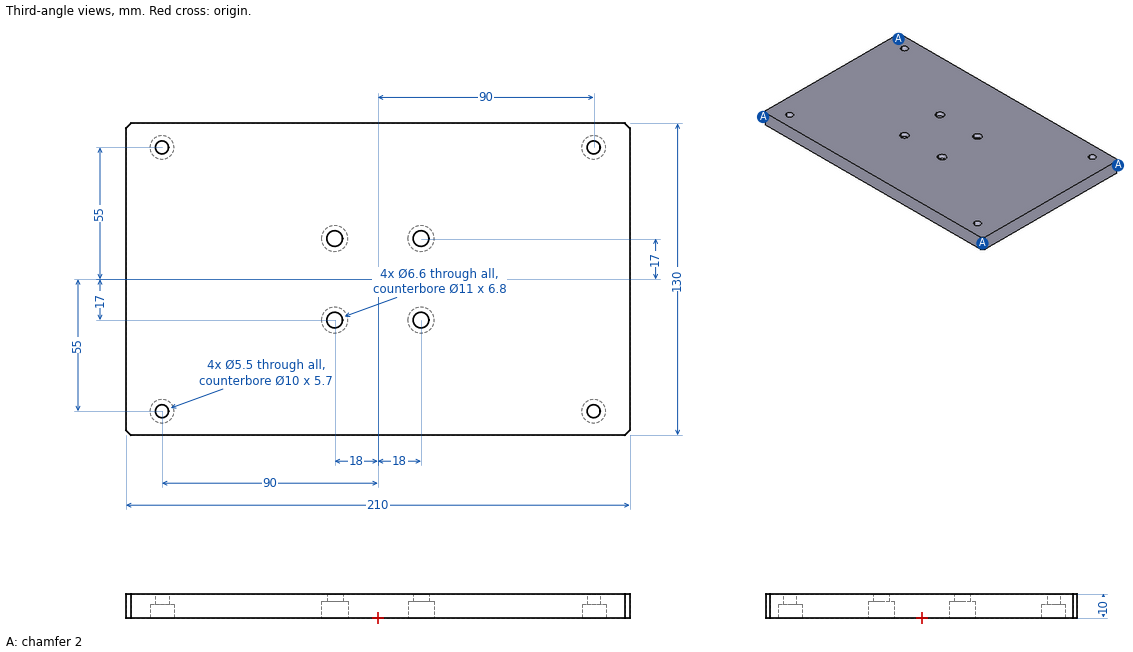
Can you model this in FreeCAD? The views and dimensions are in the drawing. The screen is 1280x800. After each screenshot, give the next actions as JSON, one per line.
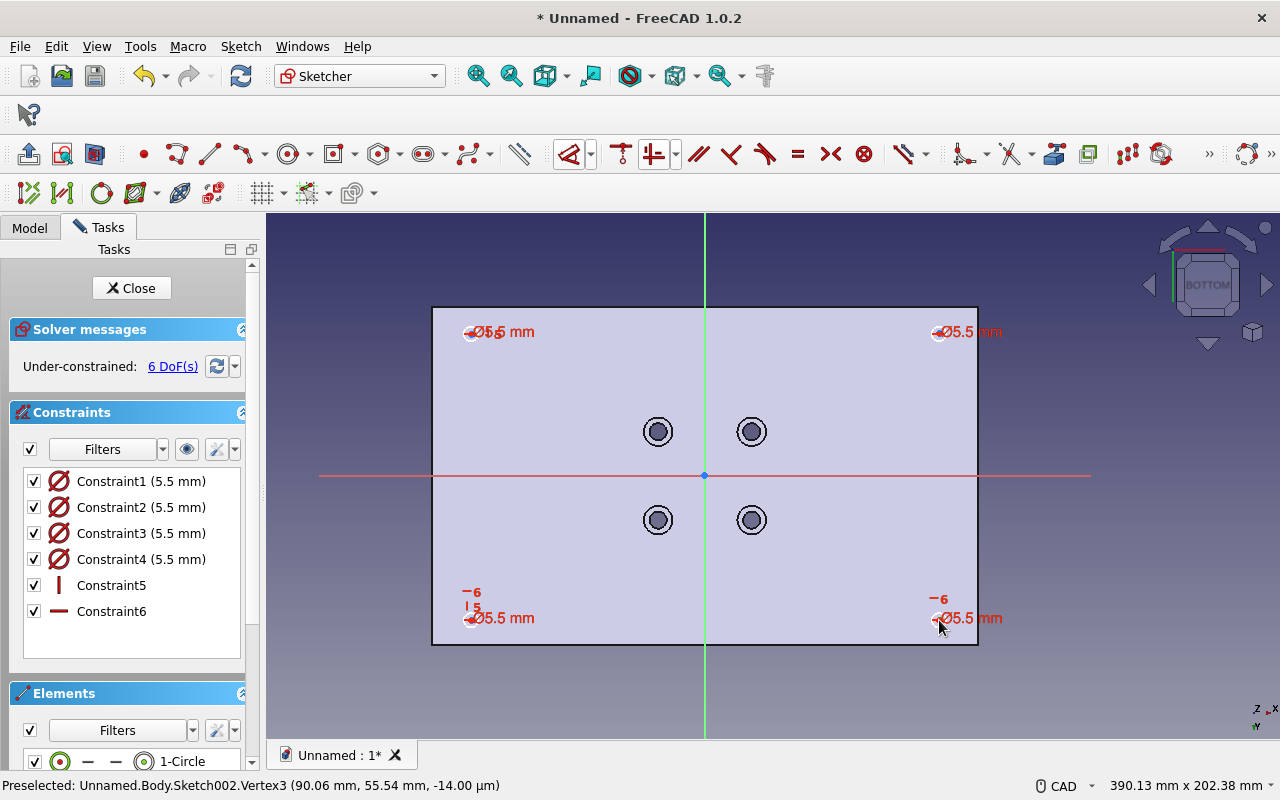
{"action": "left_click", "coordinate": [939, 334]}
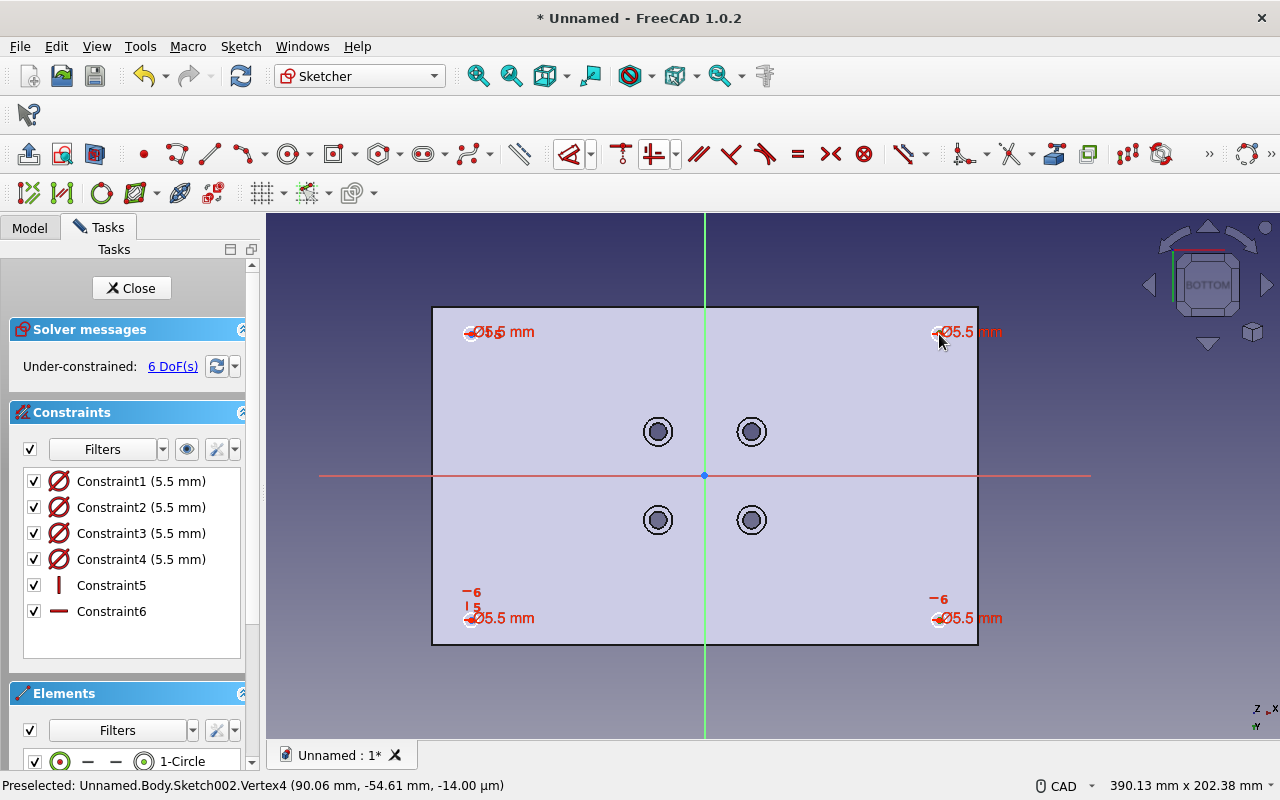
{"action": "key", "text": "v"}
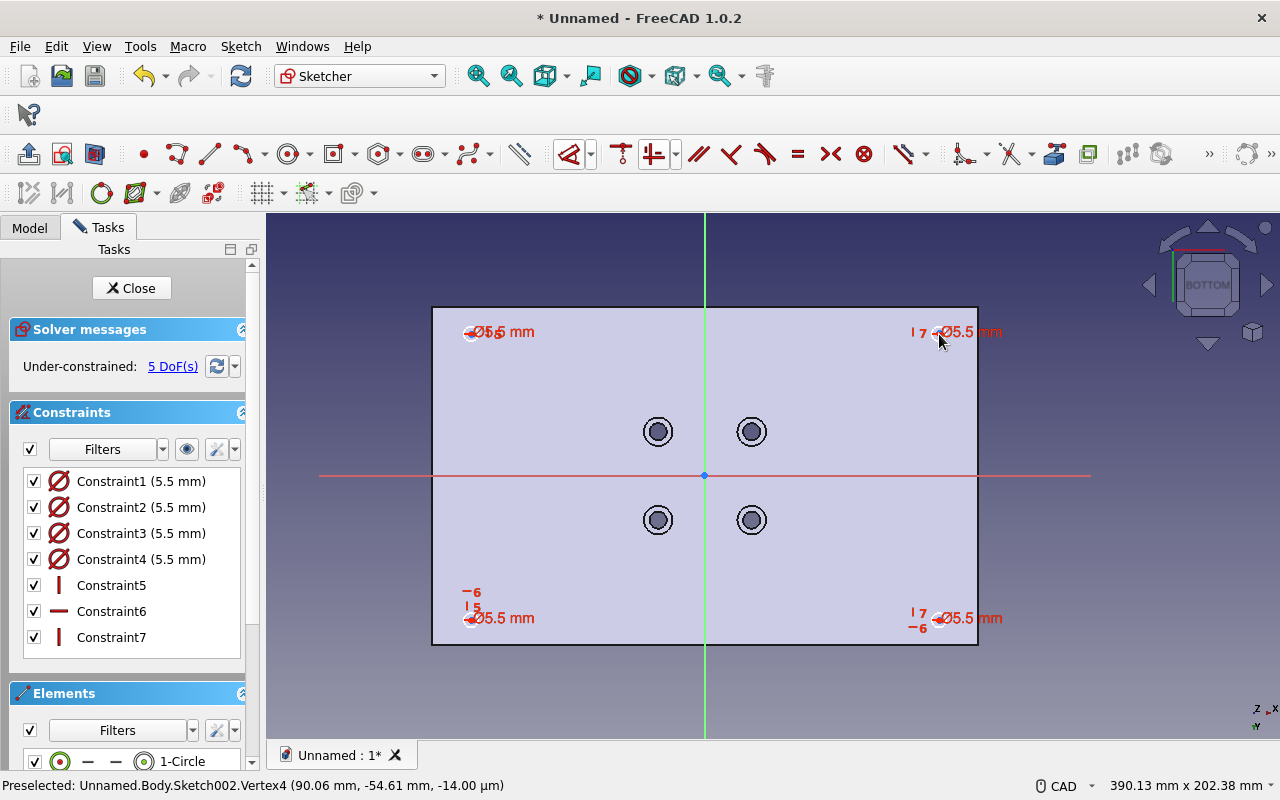
{"action": "left_click", "coordinate": [471, 334]}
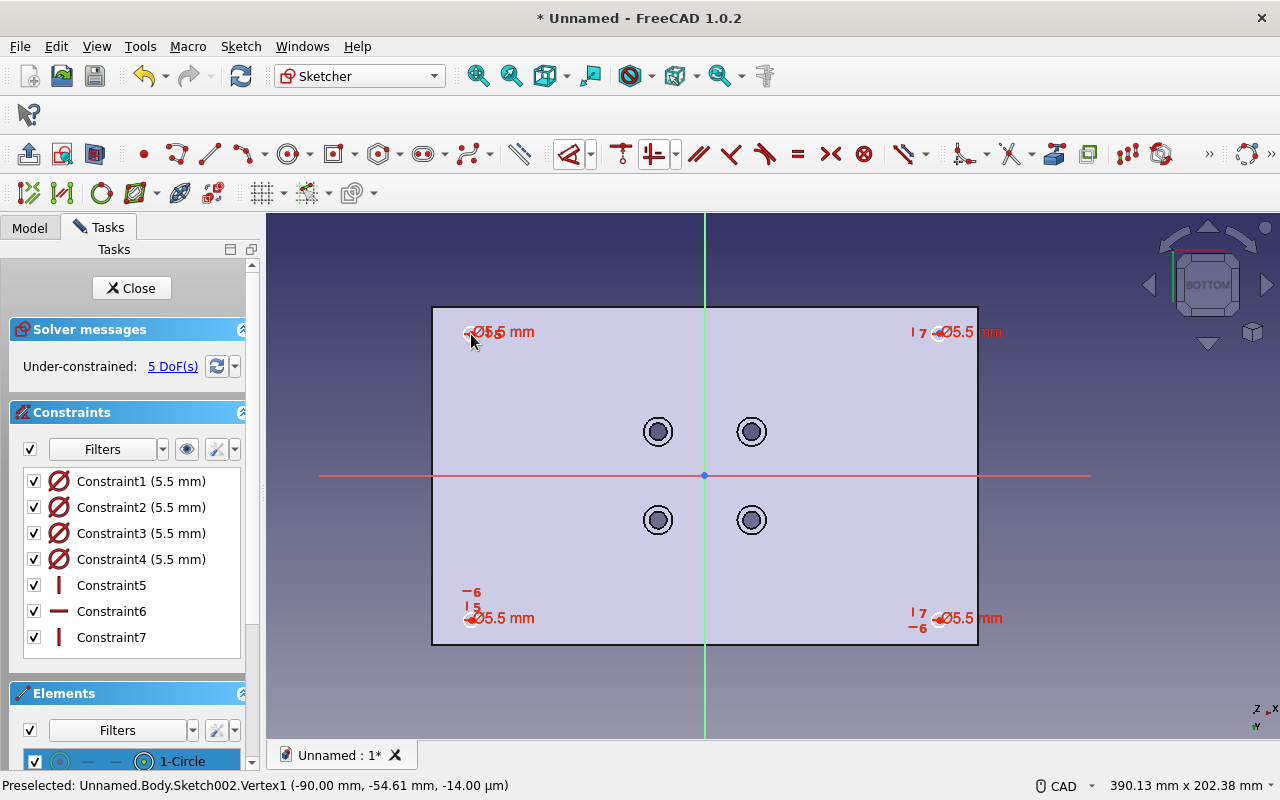
{"action": "left_click", "coordinate": [939, 334]}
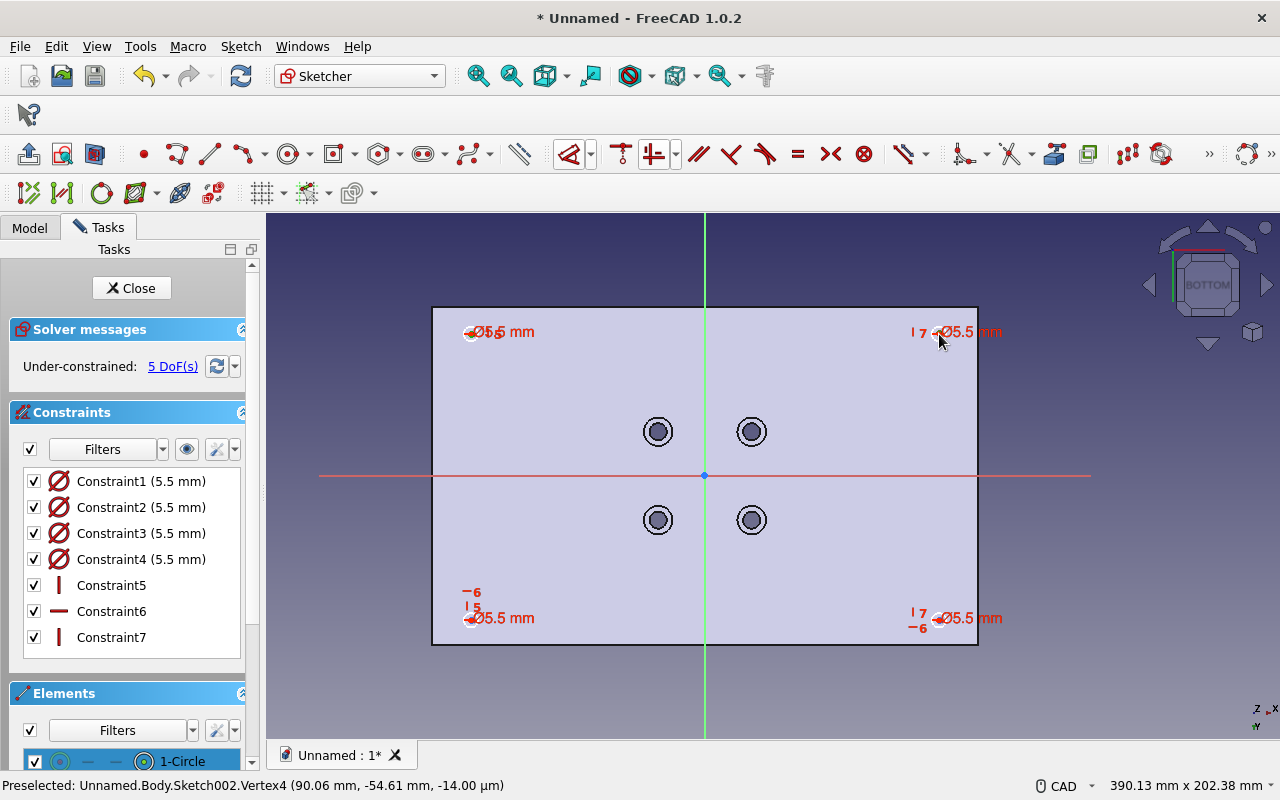
{"action": "key", "text": "h"}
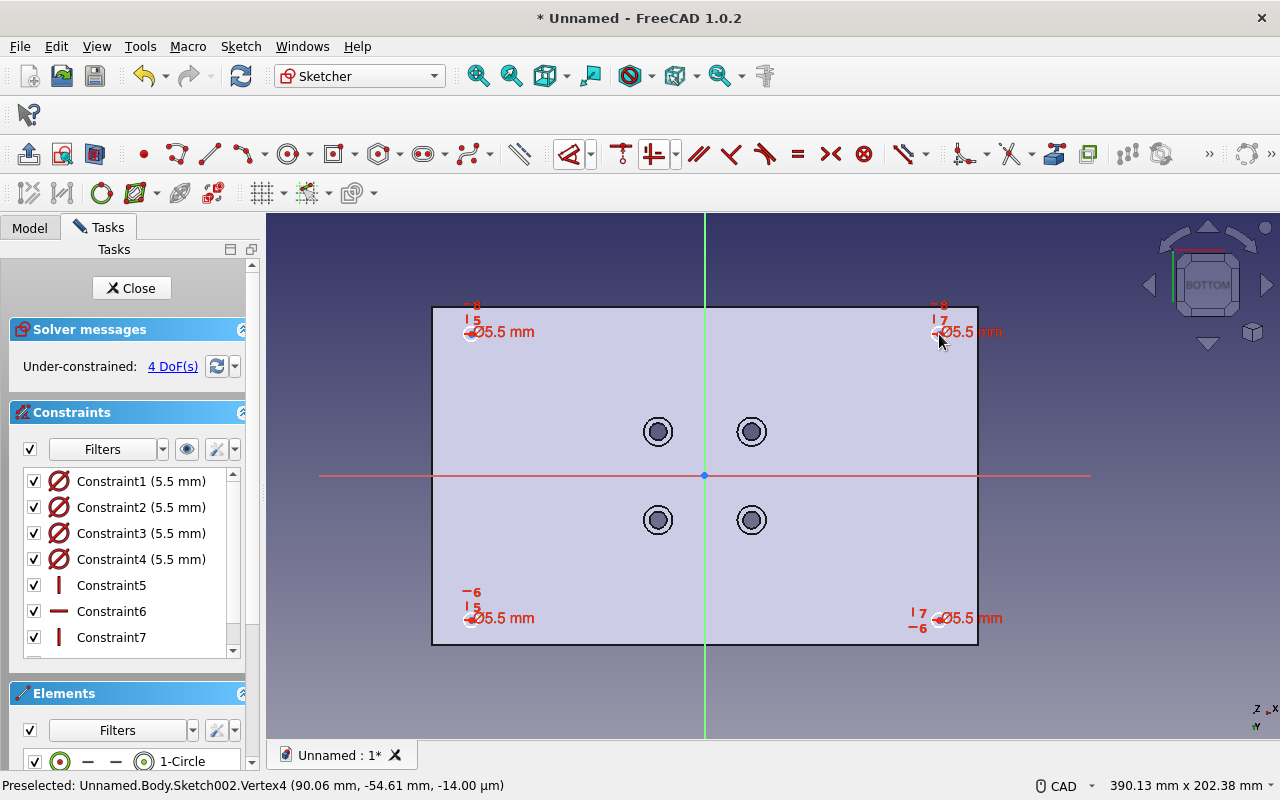
{"action": "key", "text": "d"}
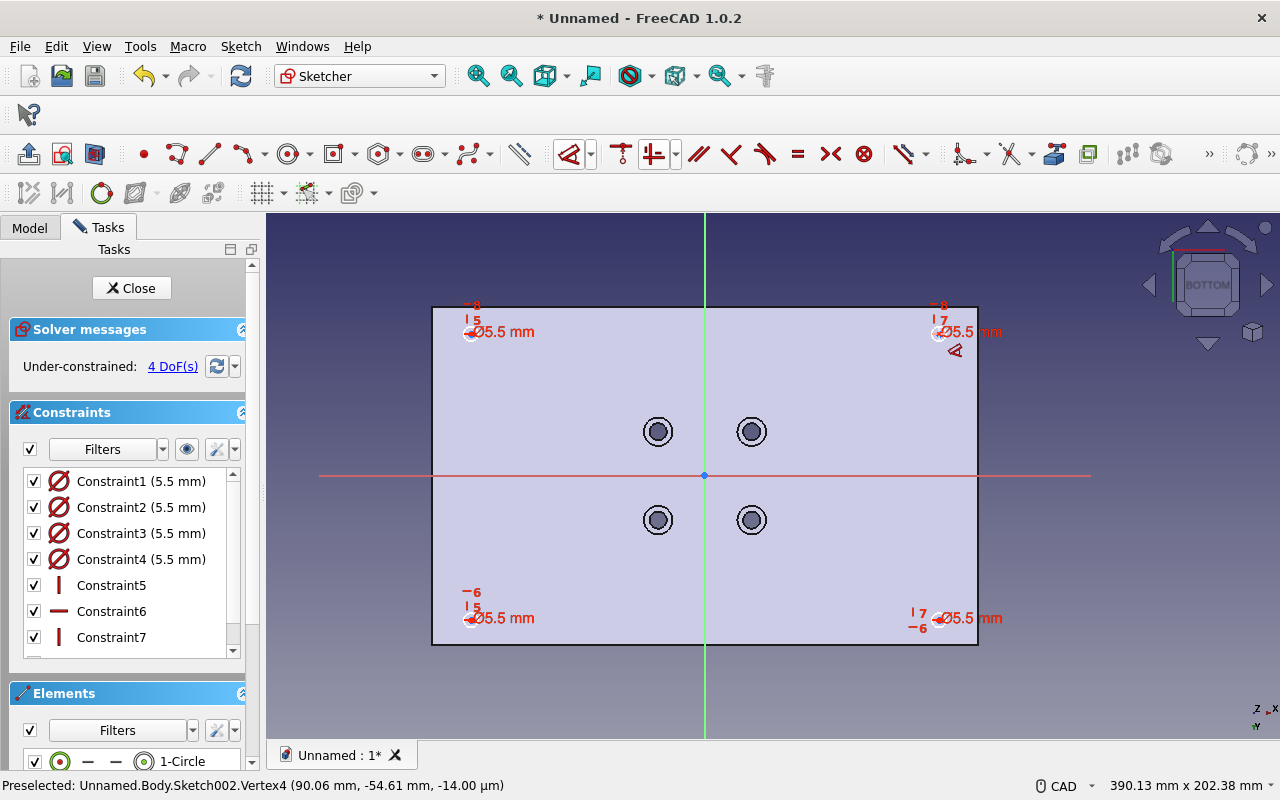
{"action": "left_click", "coordinate": [471, 334]}
{"action": "left_click", "coordinate": [588, 300]}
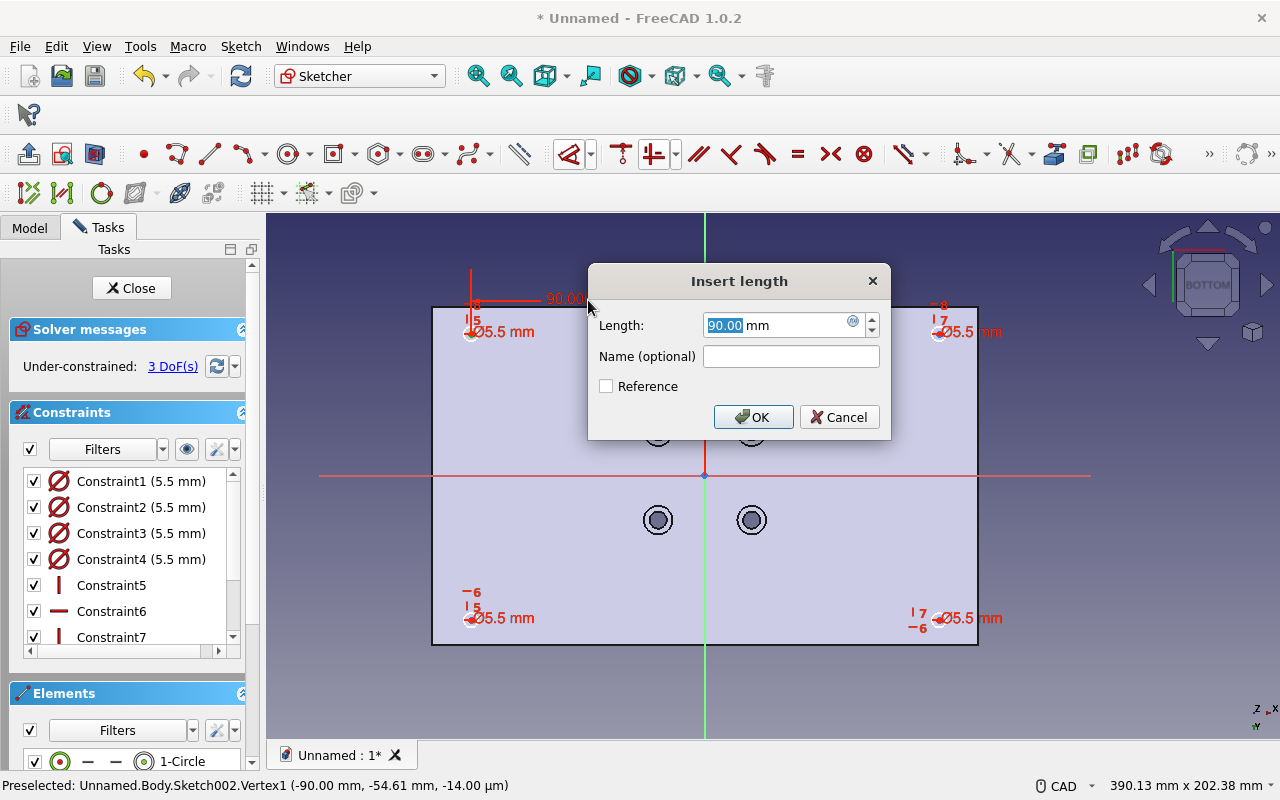
{"action": "type", "text": "90"}
{"action": "key", "text": "Return"}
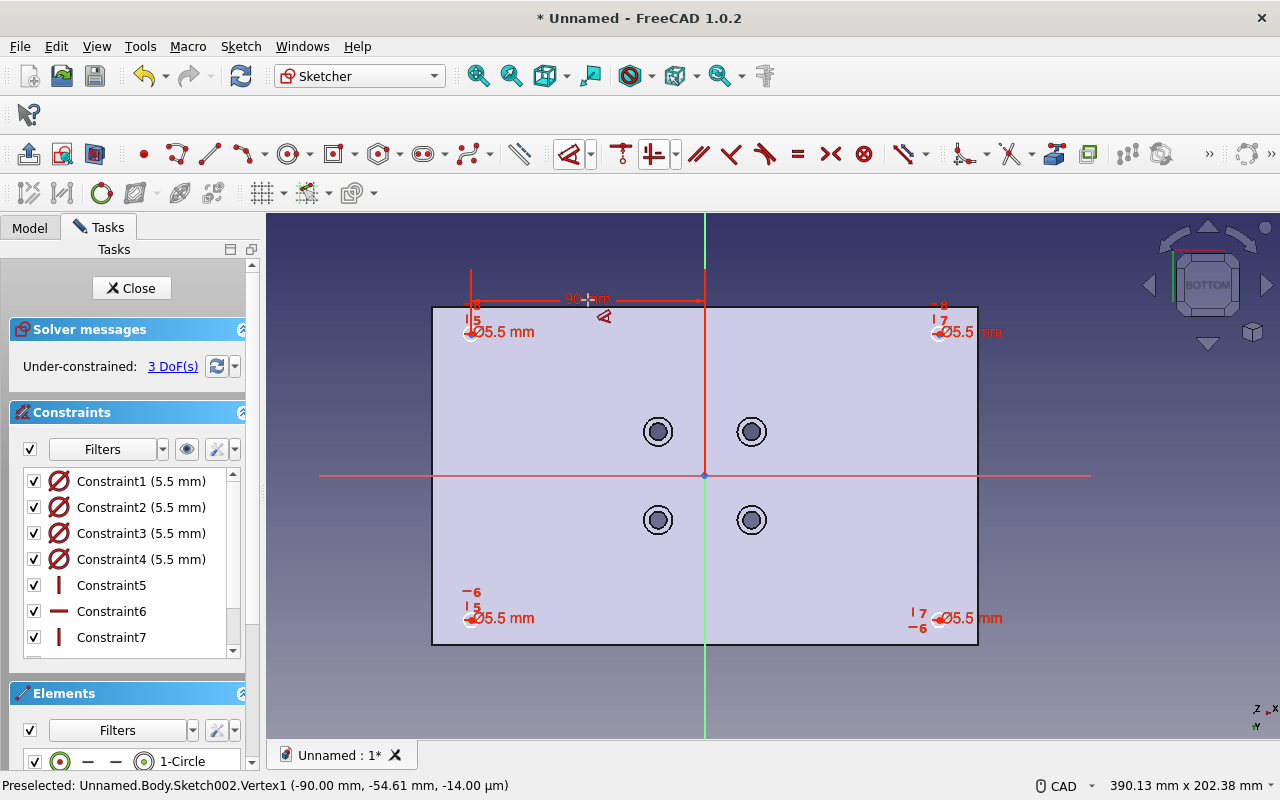
{"action": "left_click", "coordinate": [471, 334]}
{"action": "left_click", "coordinate": [437, 405]}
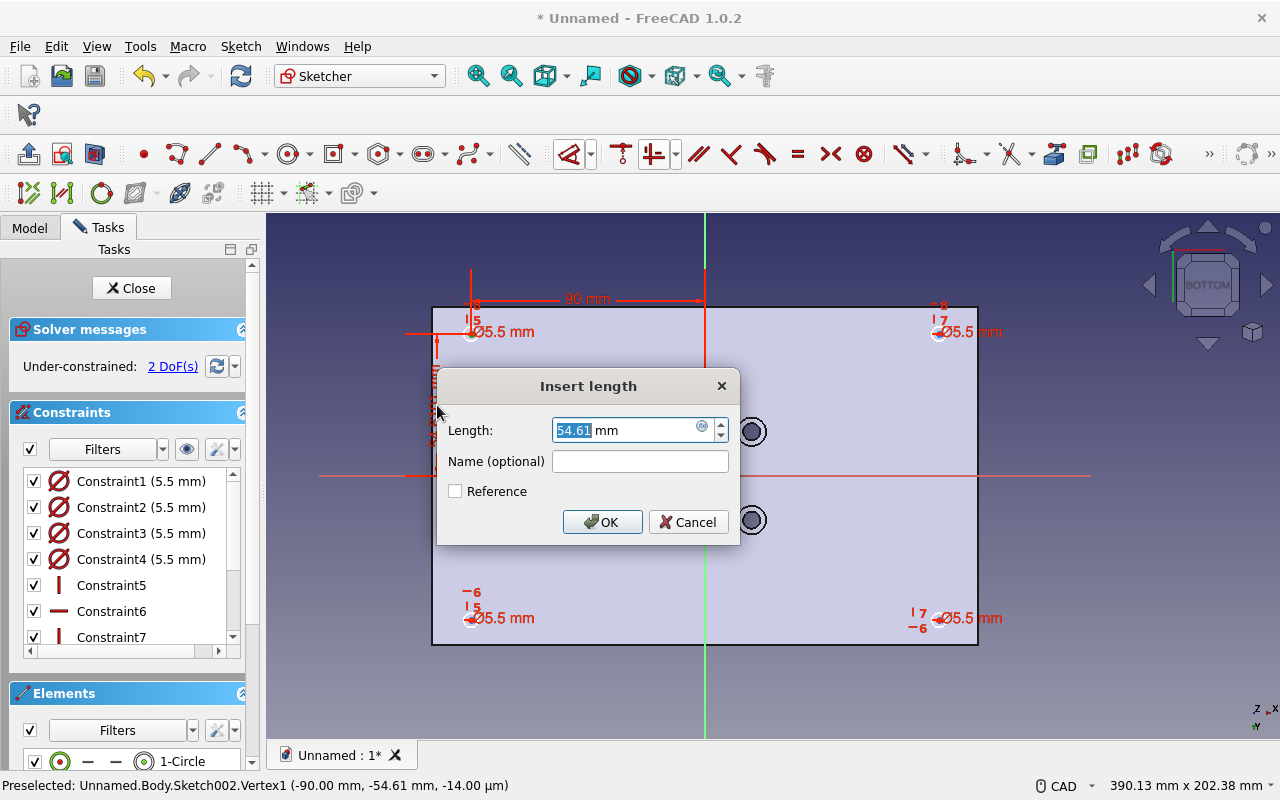
{"action": "type", "text": "55"}
{"action": "key", "text": "Return"}